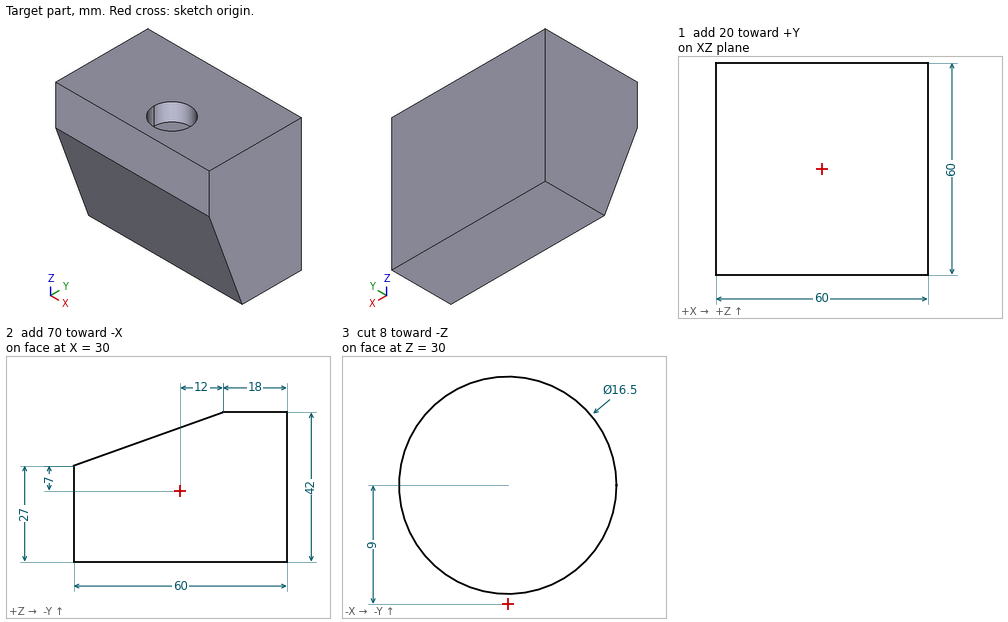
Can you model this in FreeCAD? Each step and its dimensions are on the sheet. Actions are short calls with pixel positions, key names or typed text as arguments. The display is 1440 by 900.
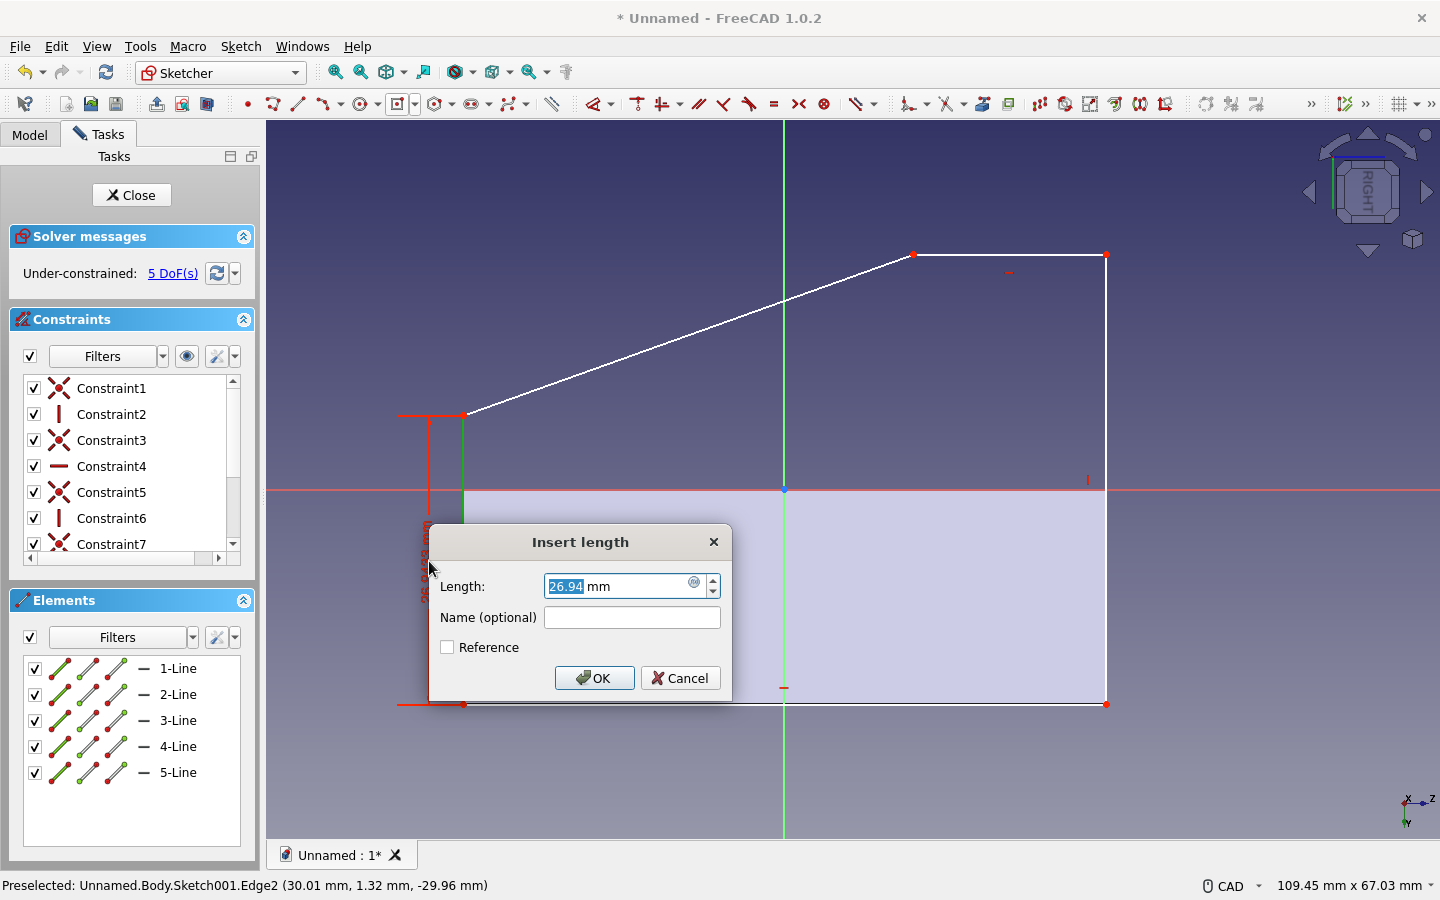
text(27)
key(Return)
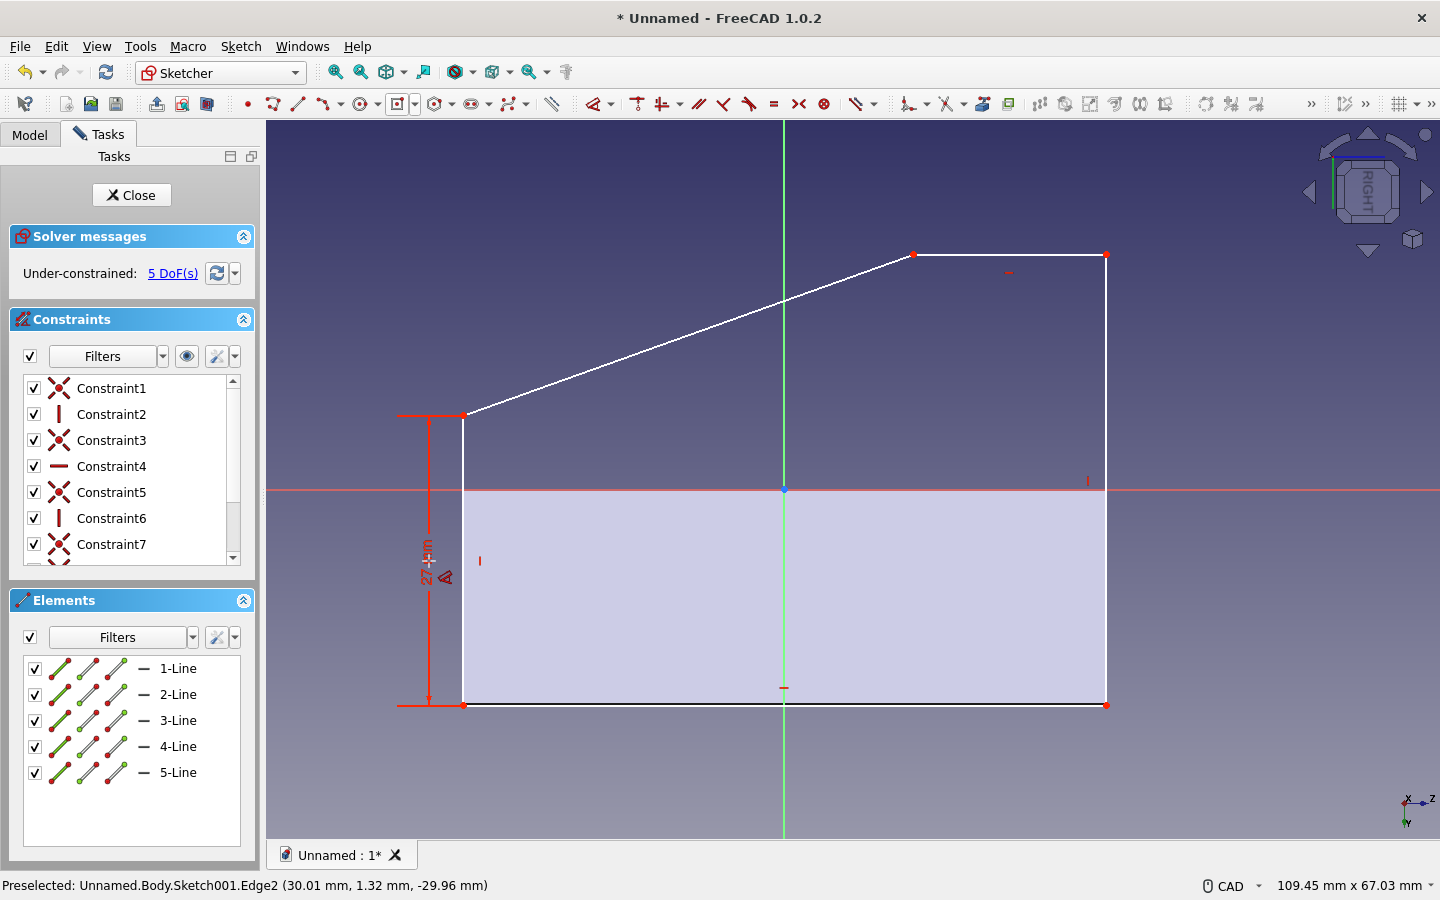
click(656, 706)
click(637, 740)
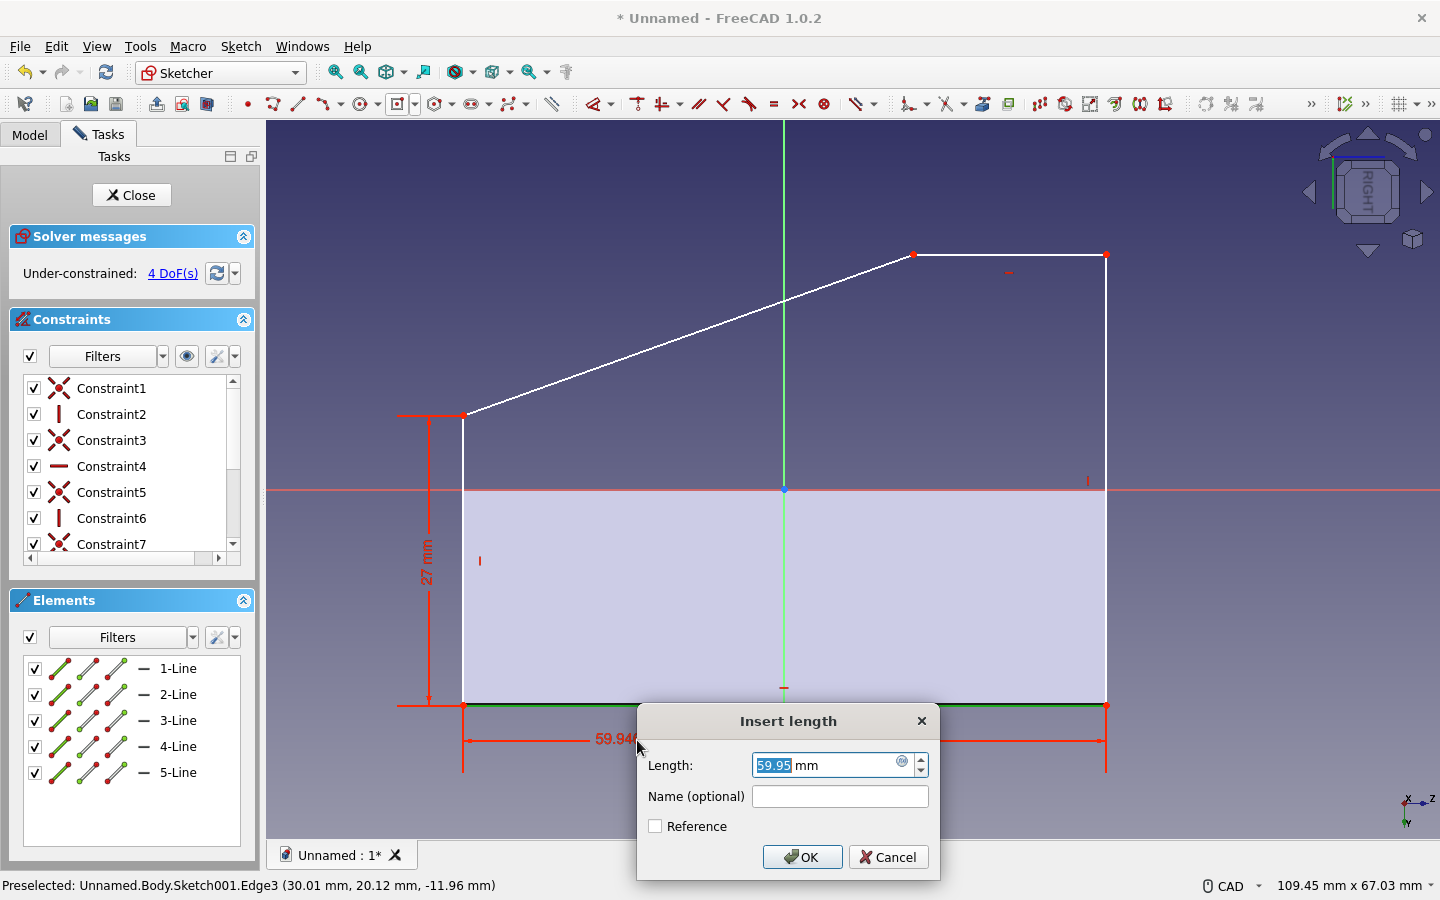
text(60)
key(Return)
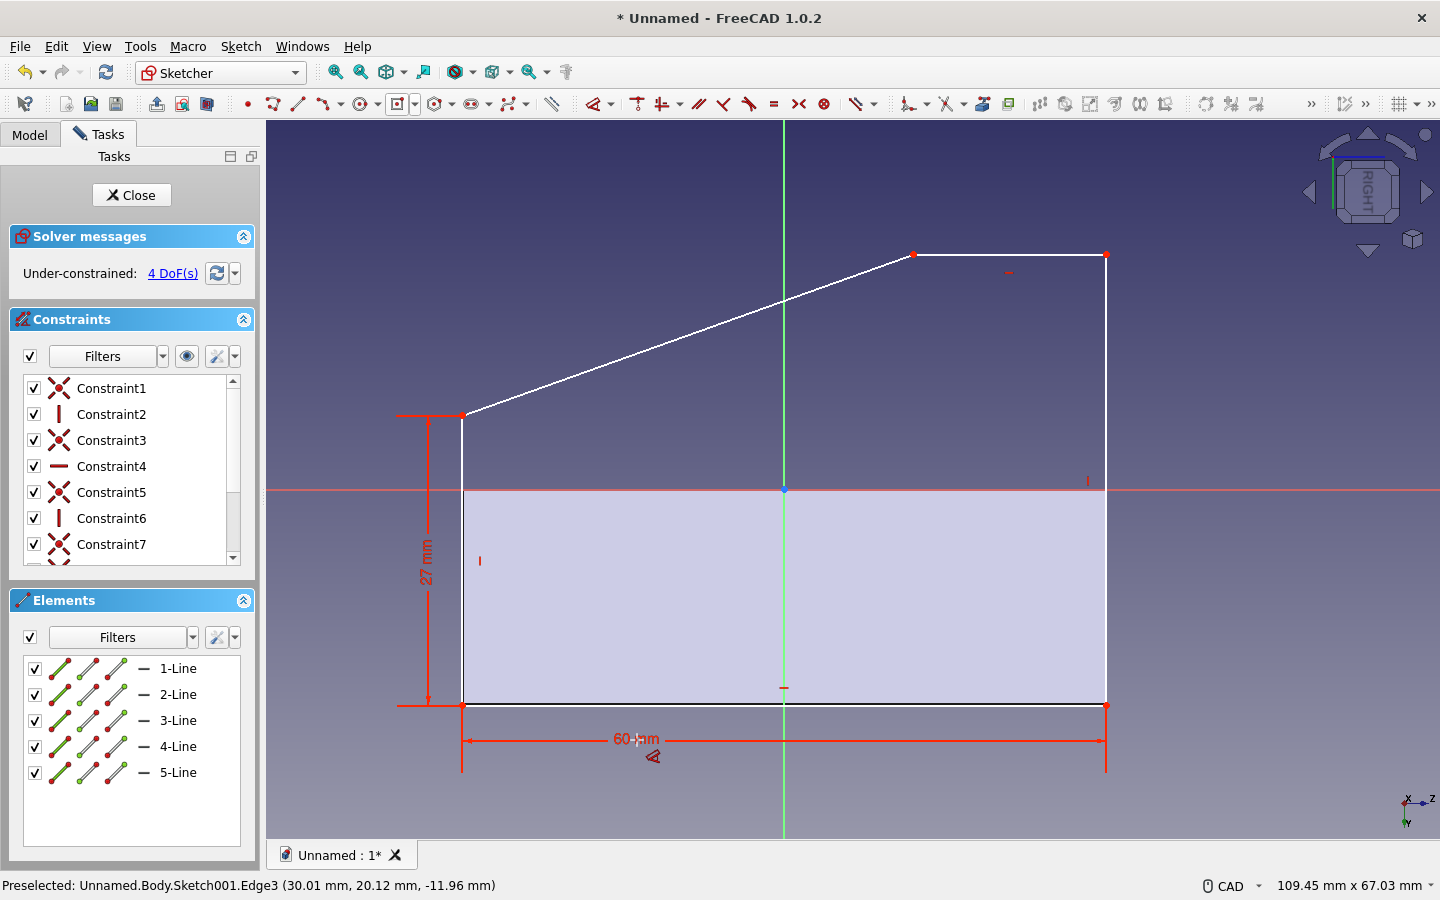
click(1106, 570)
click(1140, 377)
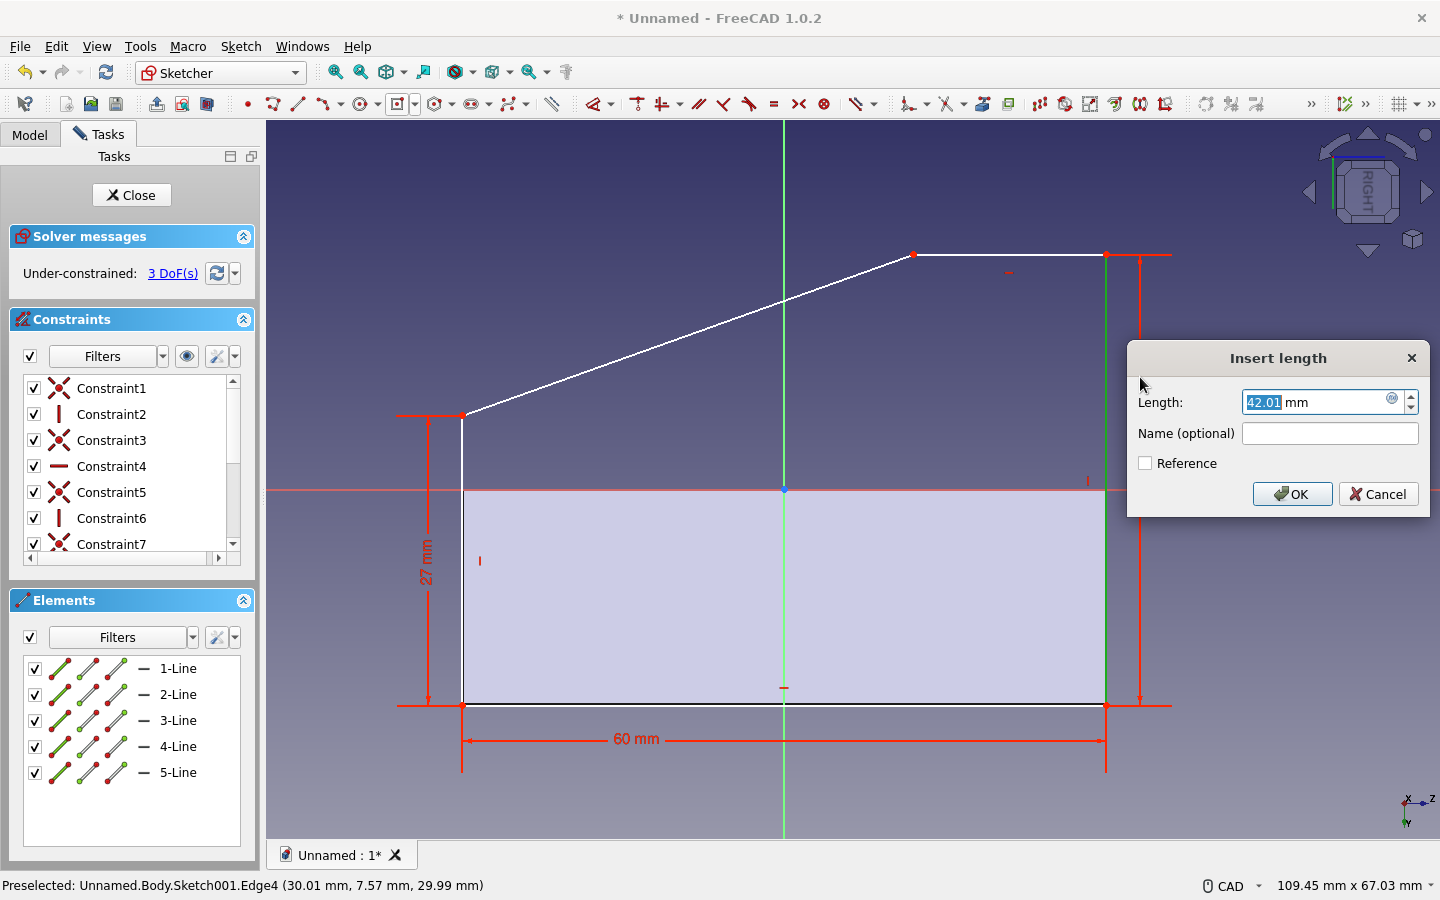
text(42)
key(Return)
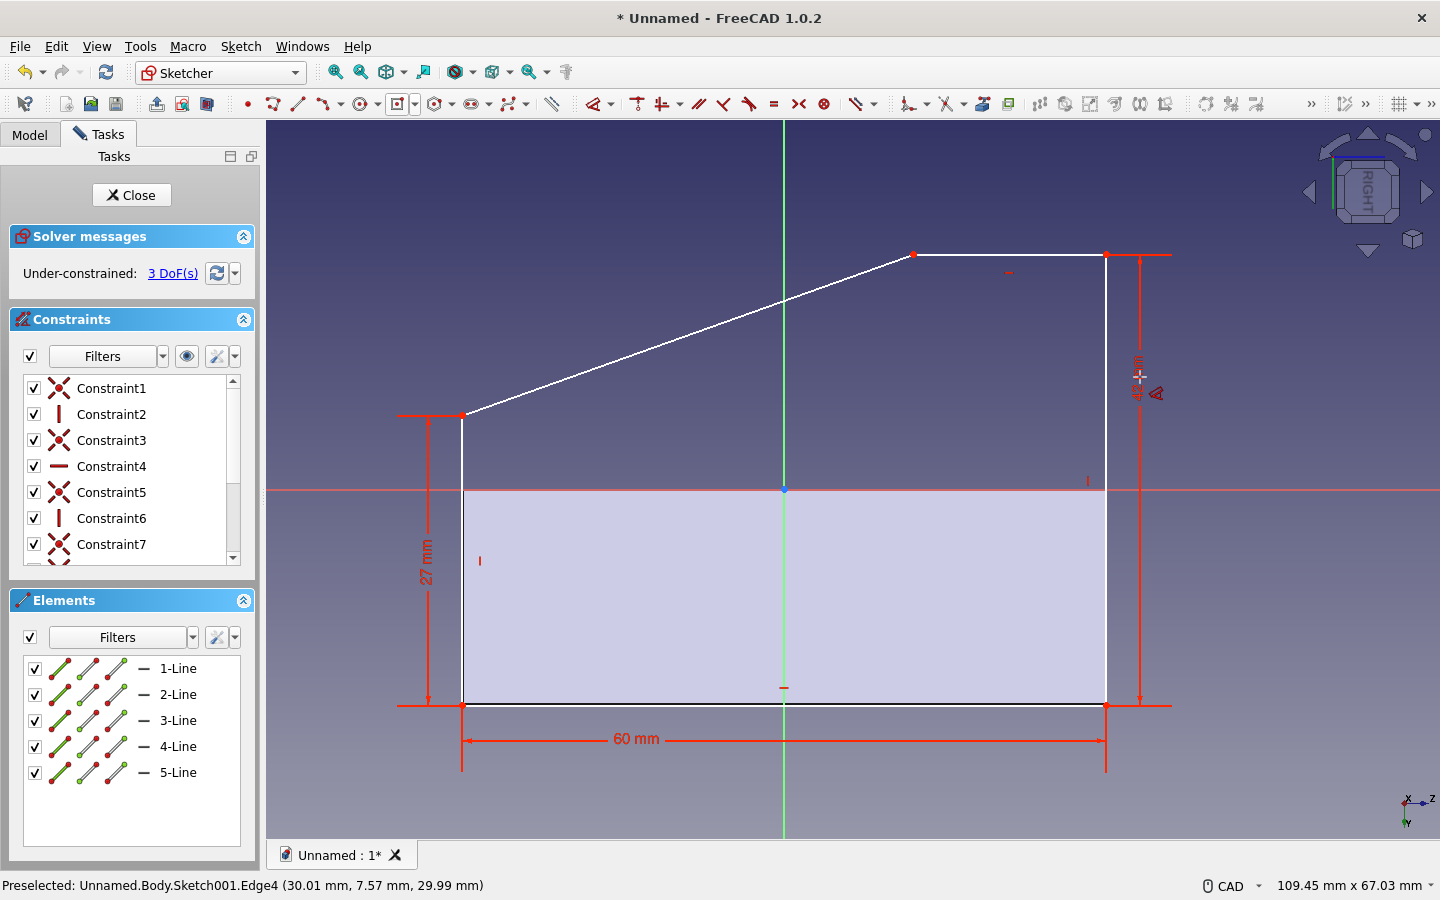
click(1048, 255)
click(1009, 221)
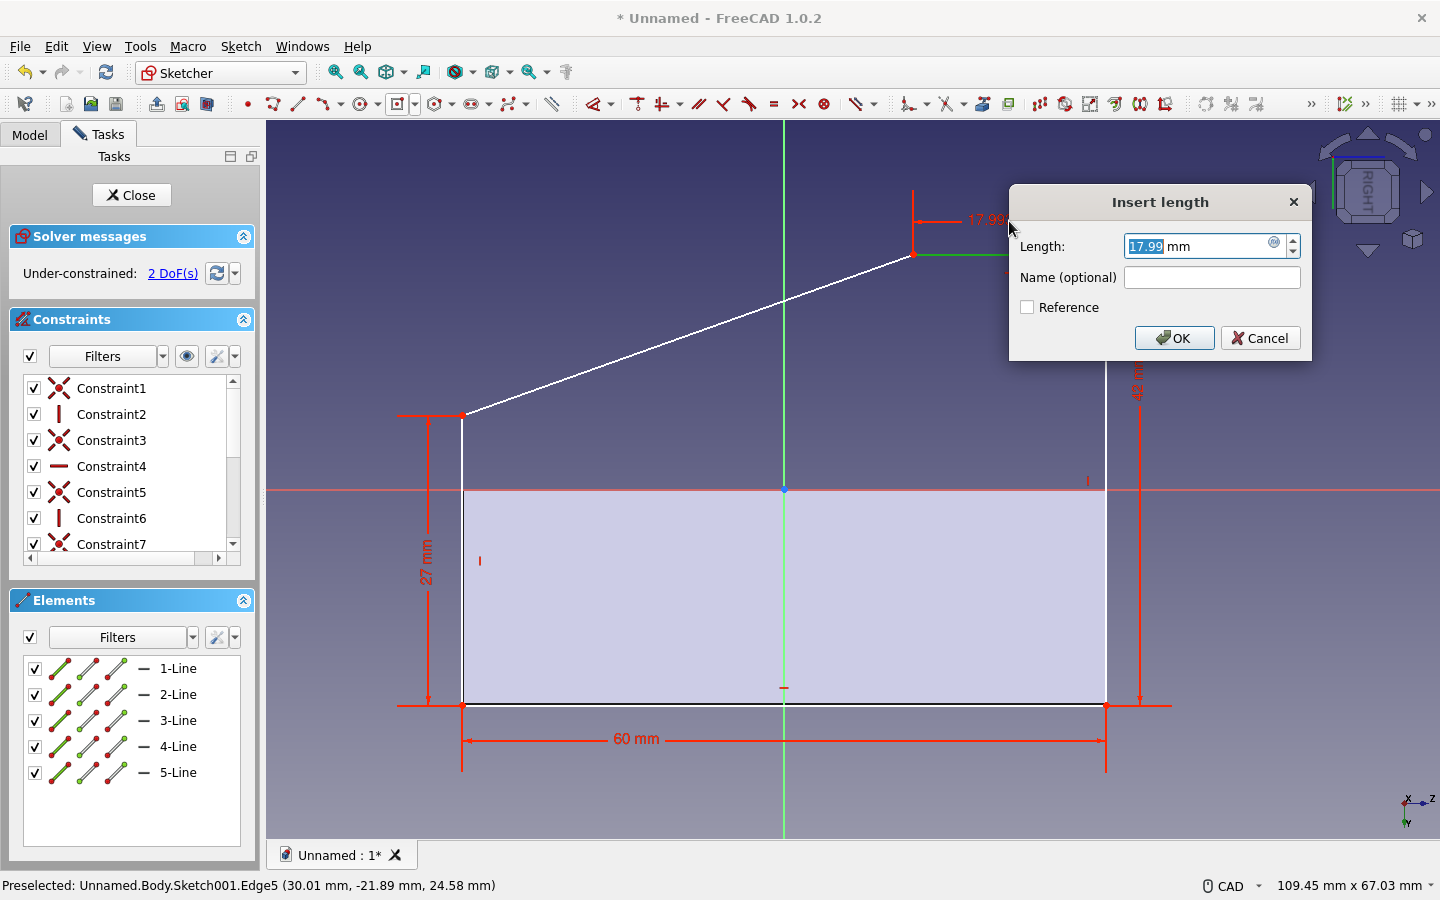
text(18)
key(Return)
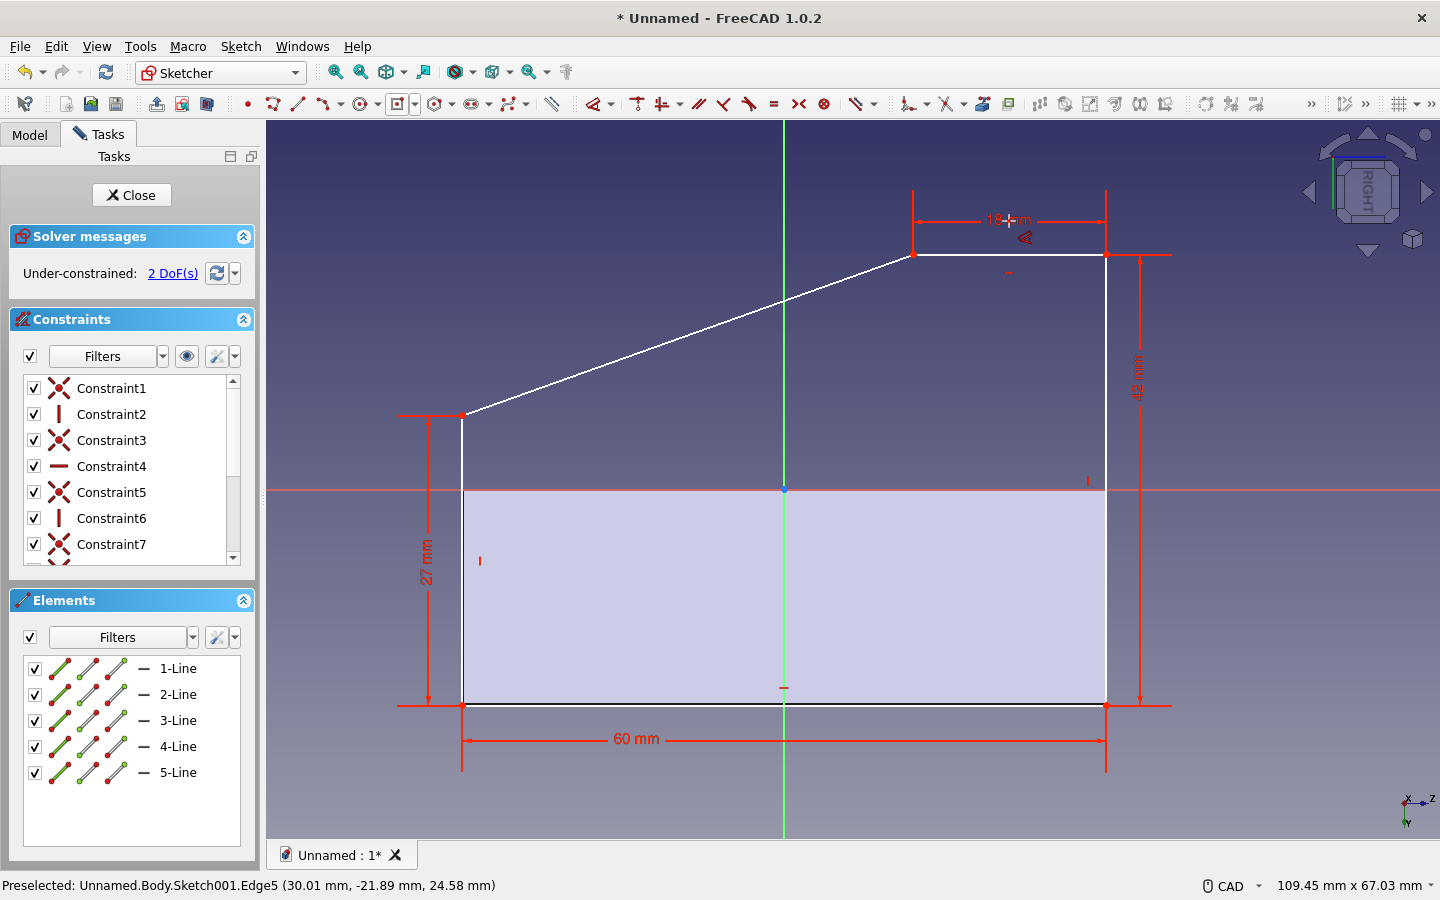
click(462, 416)
click(428, 453)